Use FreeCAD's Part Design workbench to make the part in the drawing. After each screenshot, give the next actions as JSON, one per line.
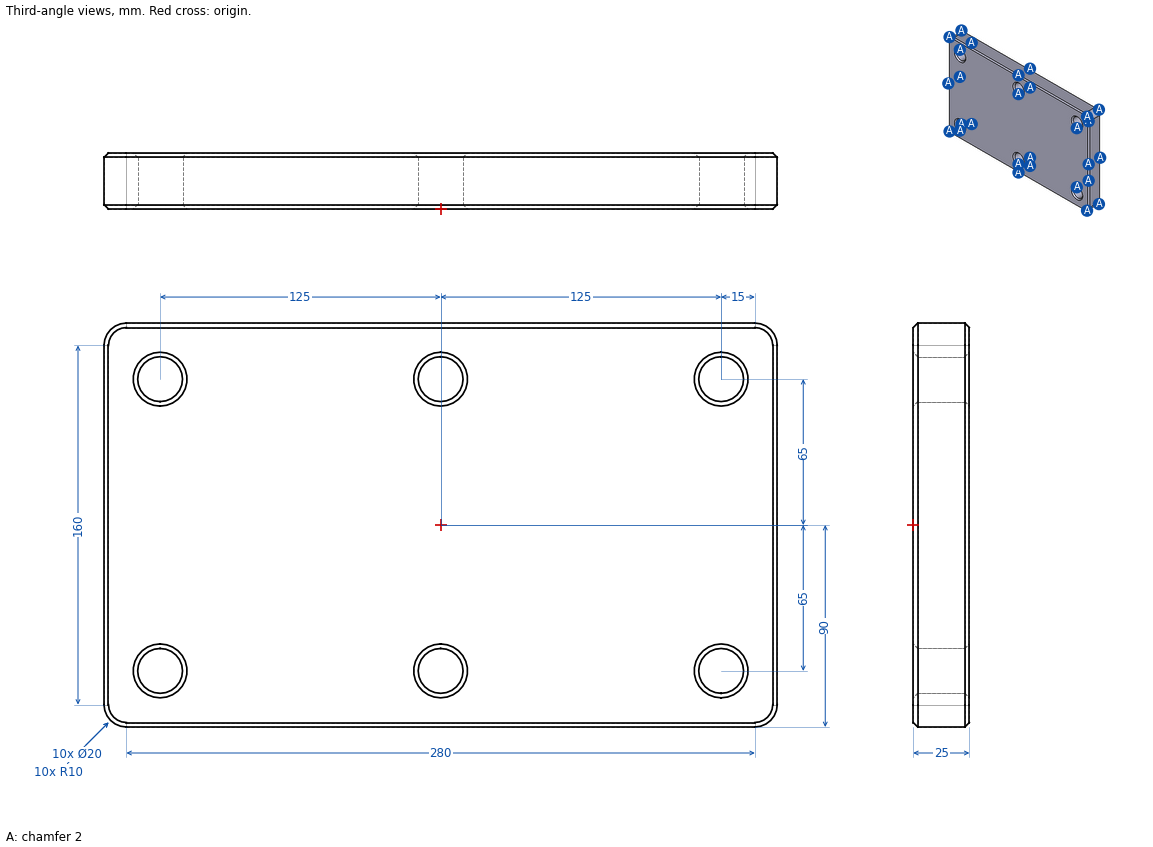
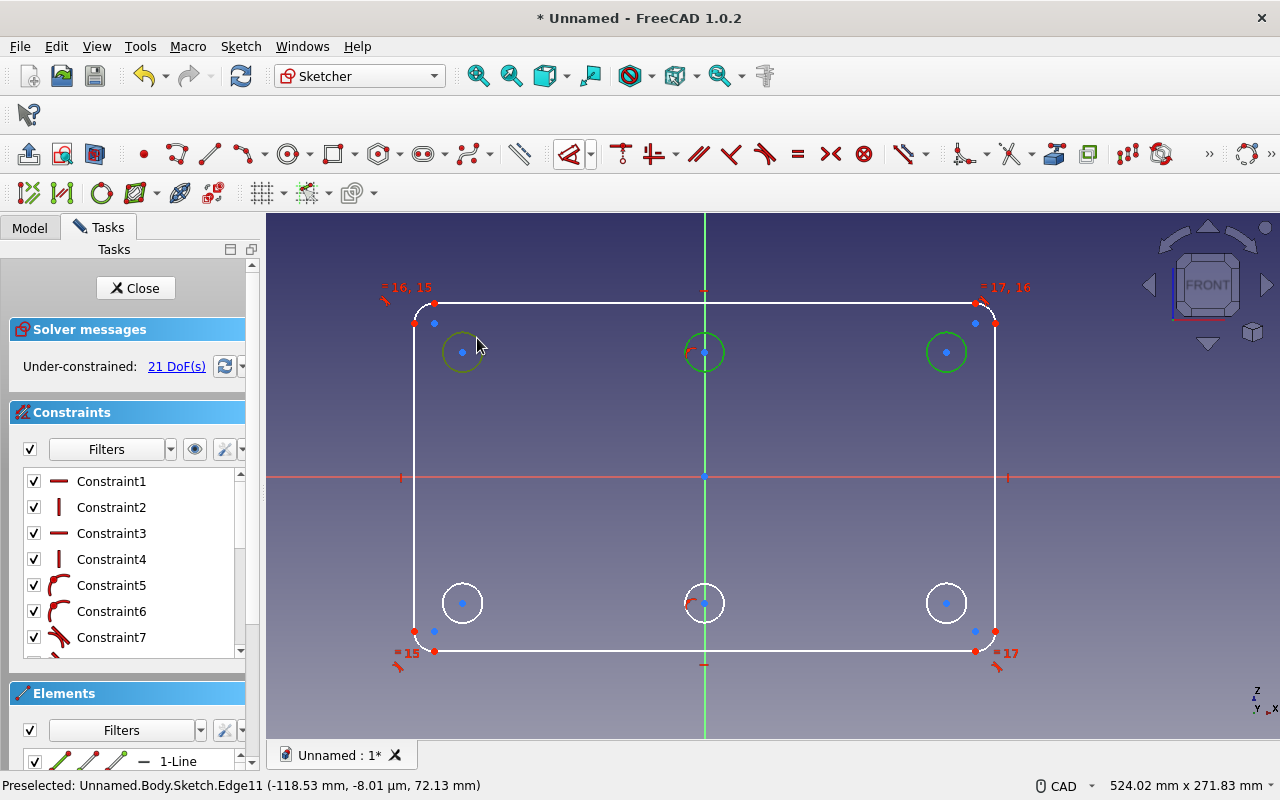
{"action": "left_click", "coordinate": [961, 589]}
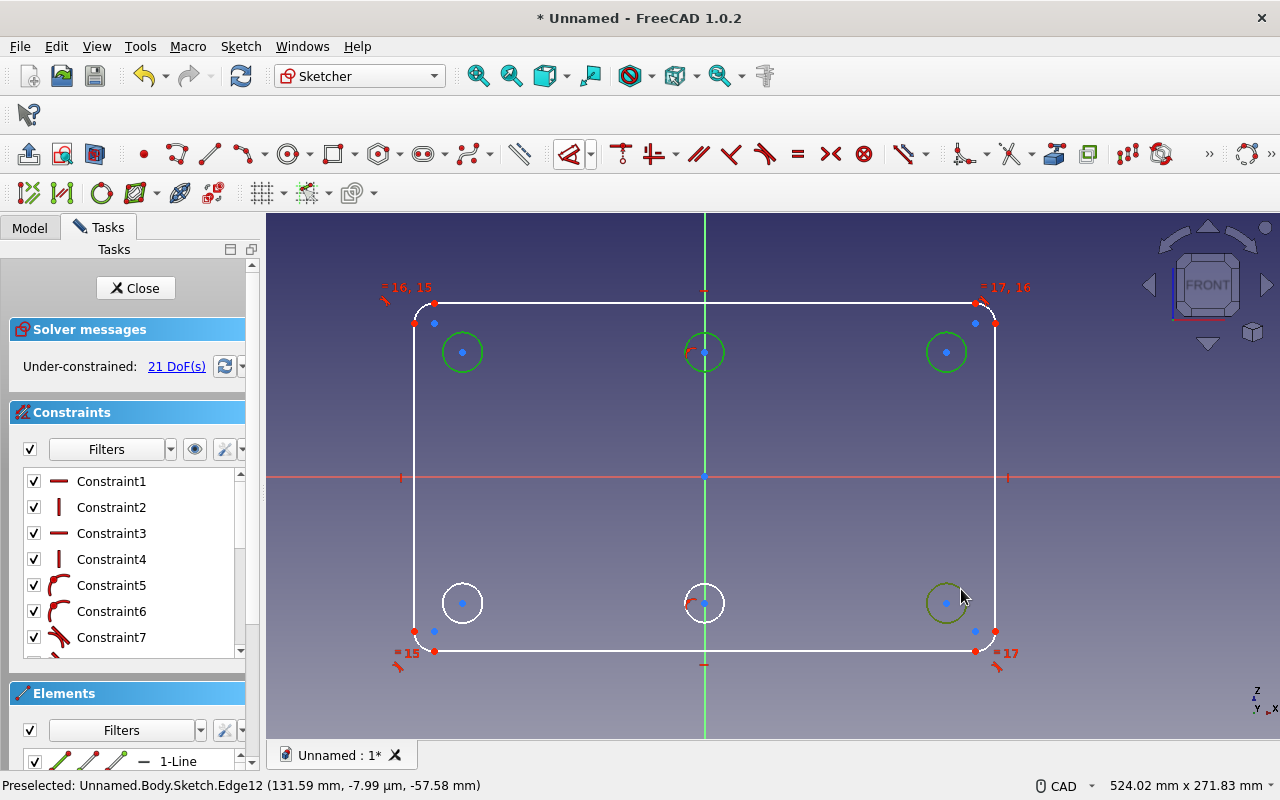
{"action": "left_click", "coordinate": [718, 590]}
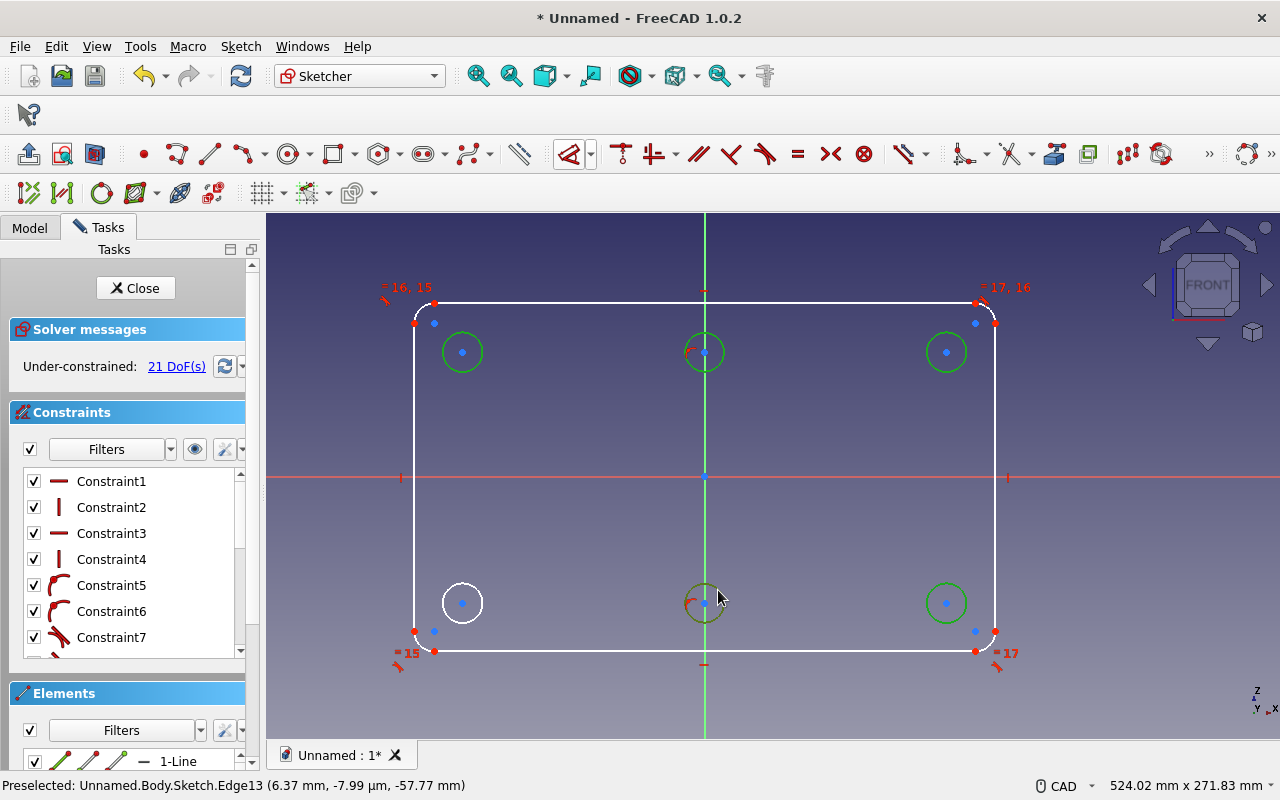
{"action": "left_click", "coordinate": [477, 589]}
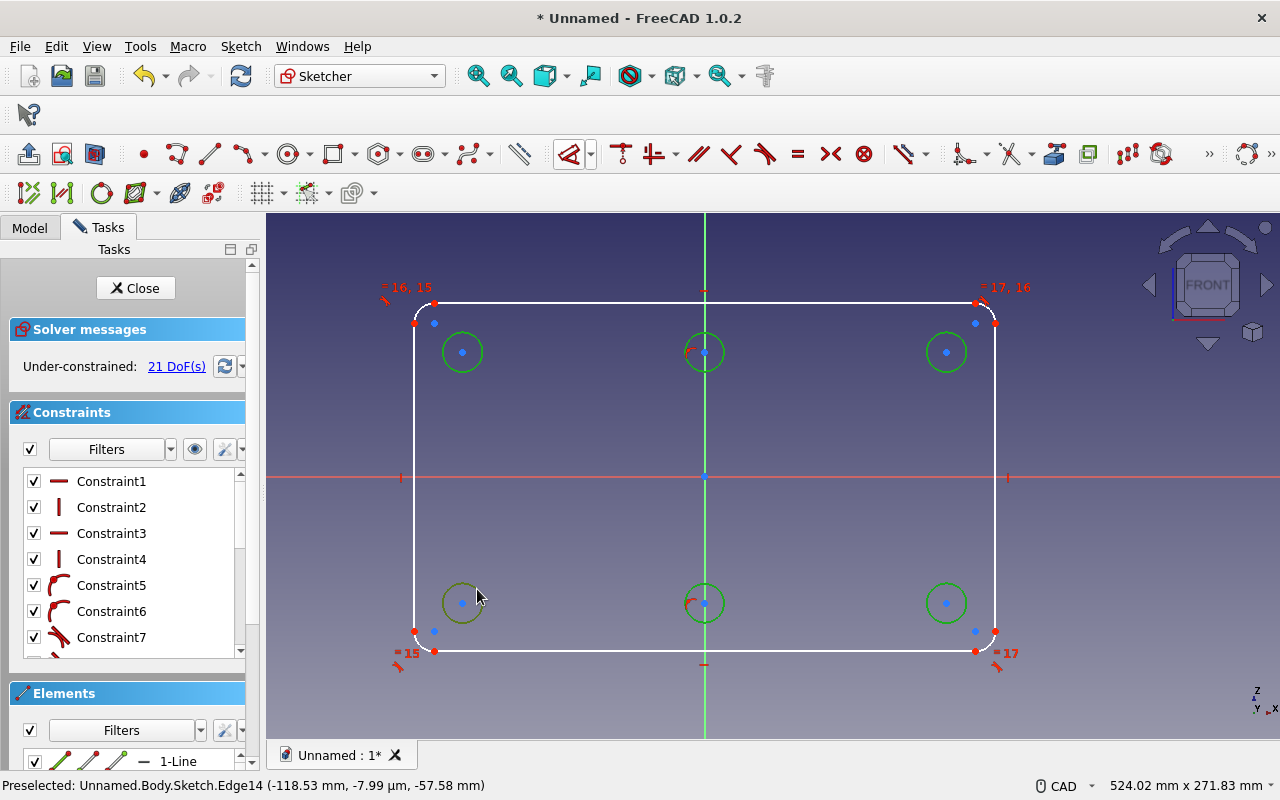
{"action": "left_click", "coordinate": [798, 154]}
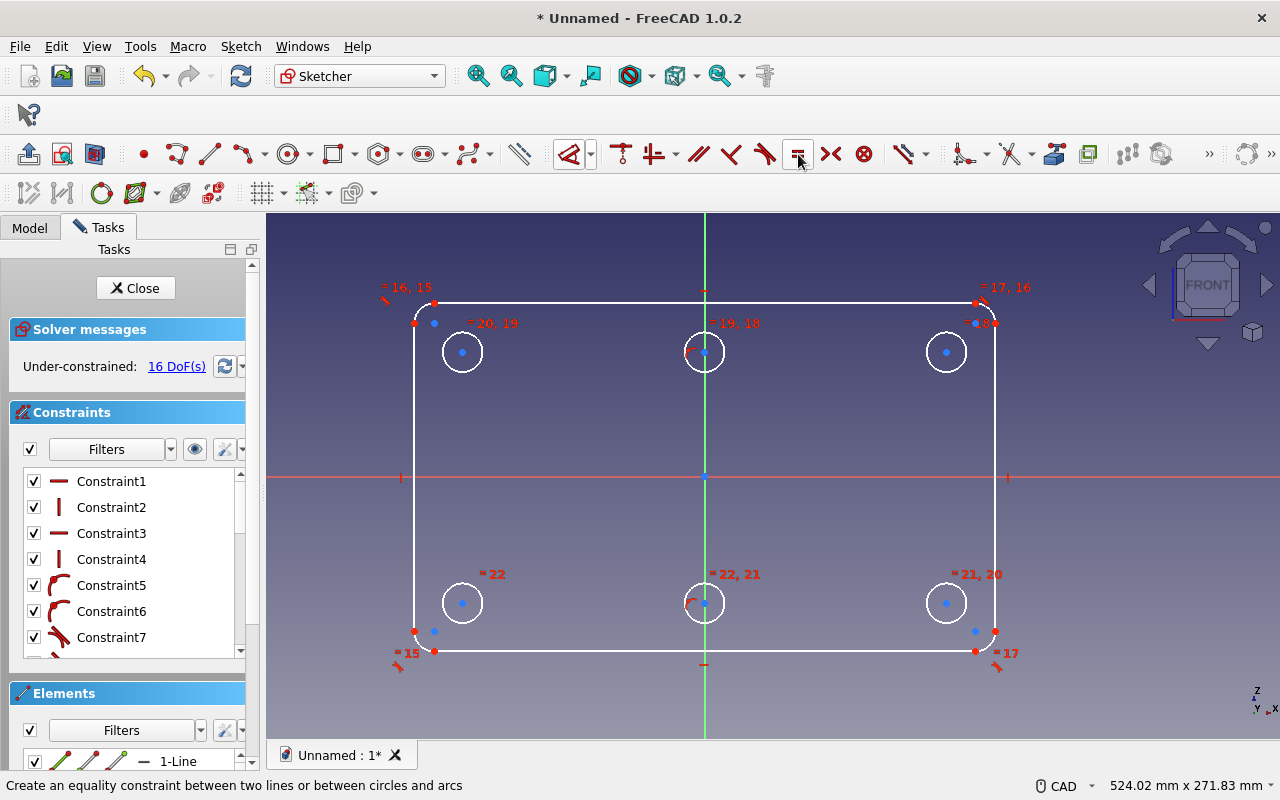
{"action": "left_click", "coordinate": [947, 352]}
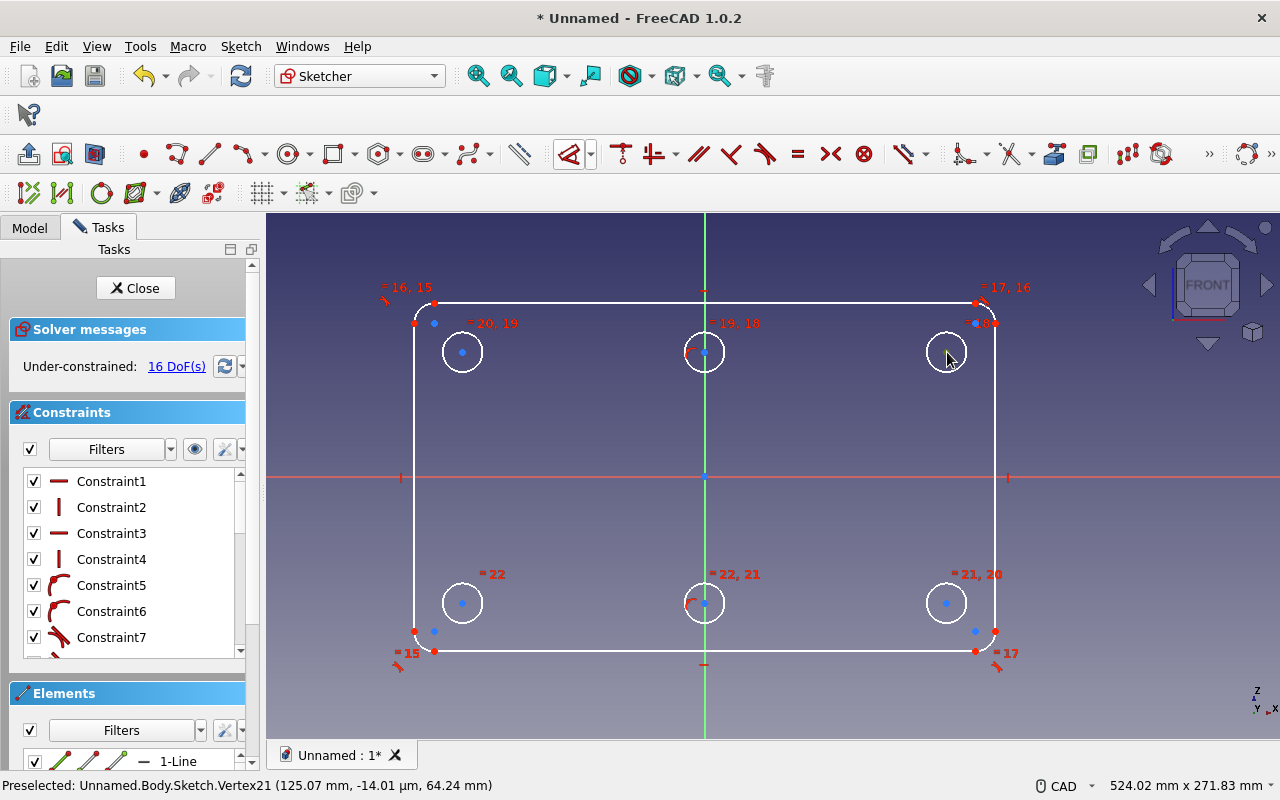
{"action": "left_click", "coordinate": [705, 352]}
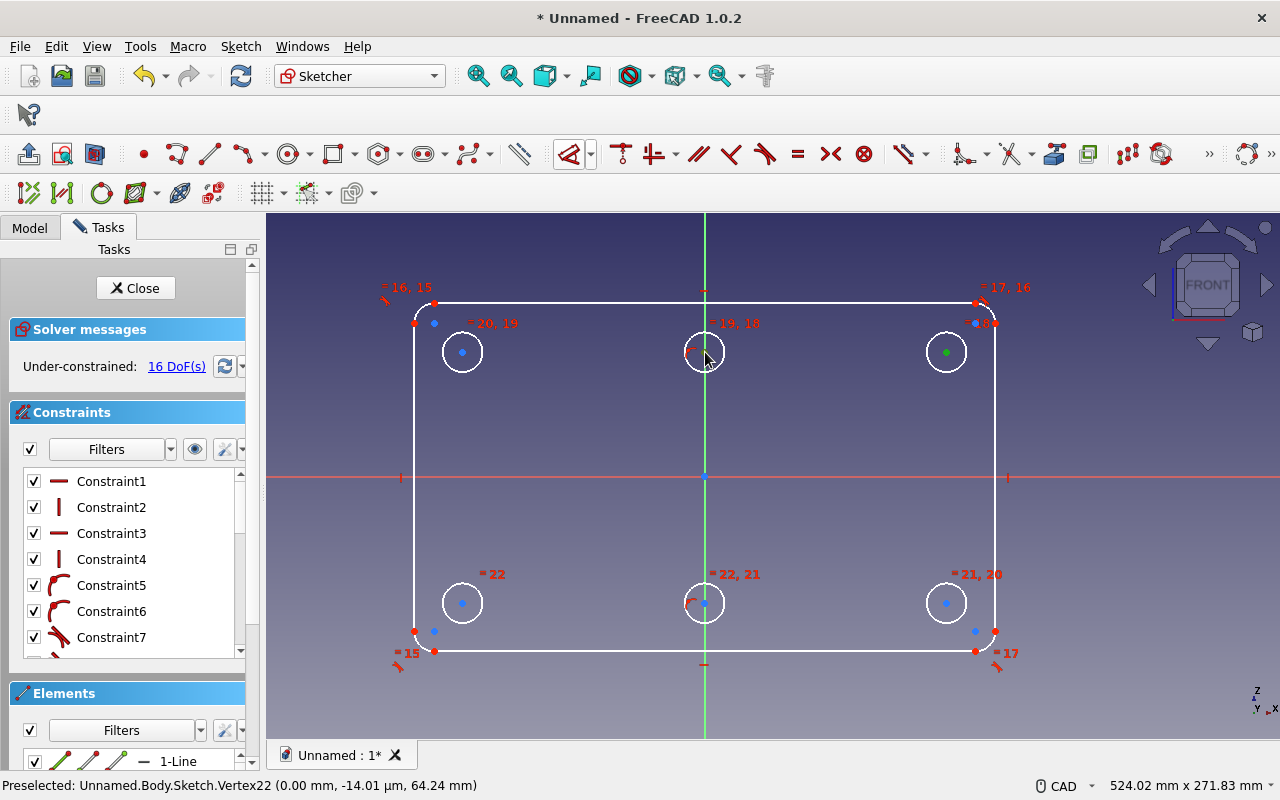
{"action": "left_click", "coordinate": [676, 154]}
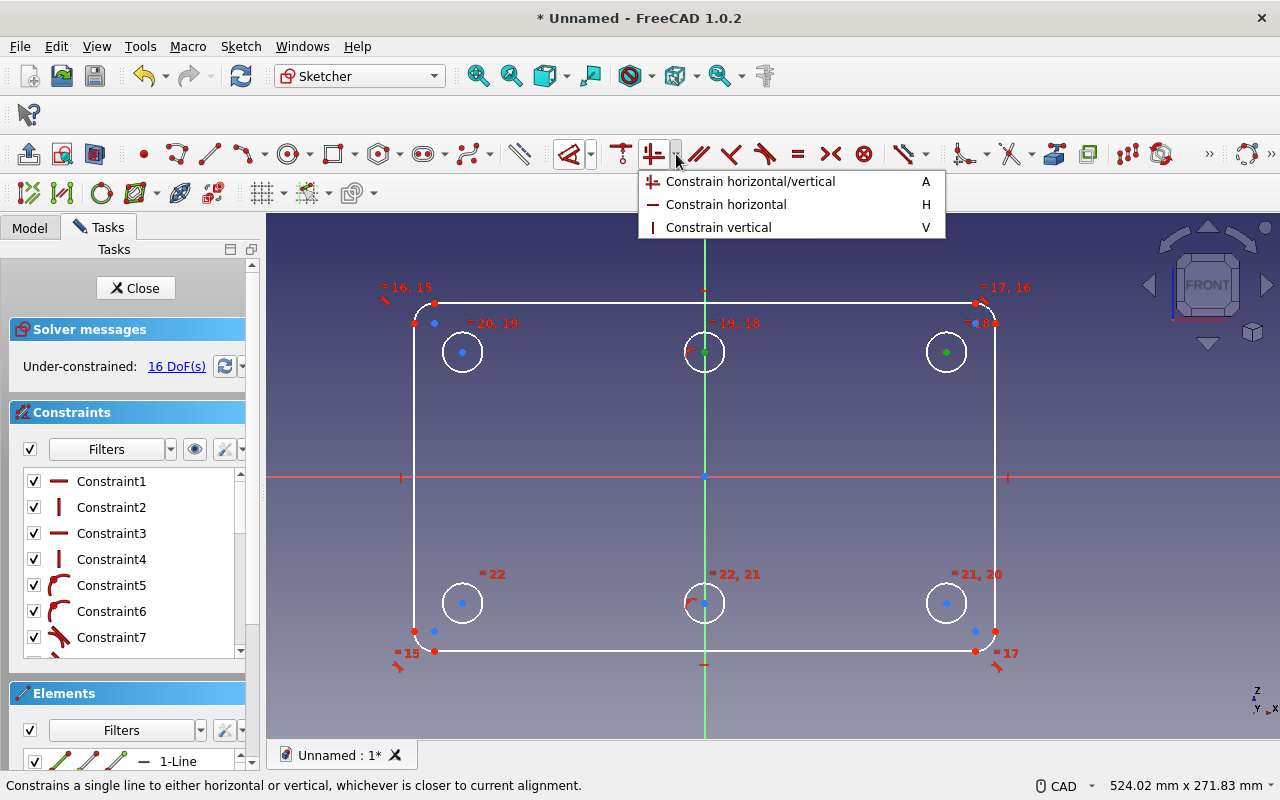
{"action": "left_click", "coordinate": [792, 204]}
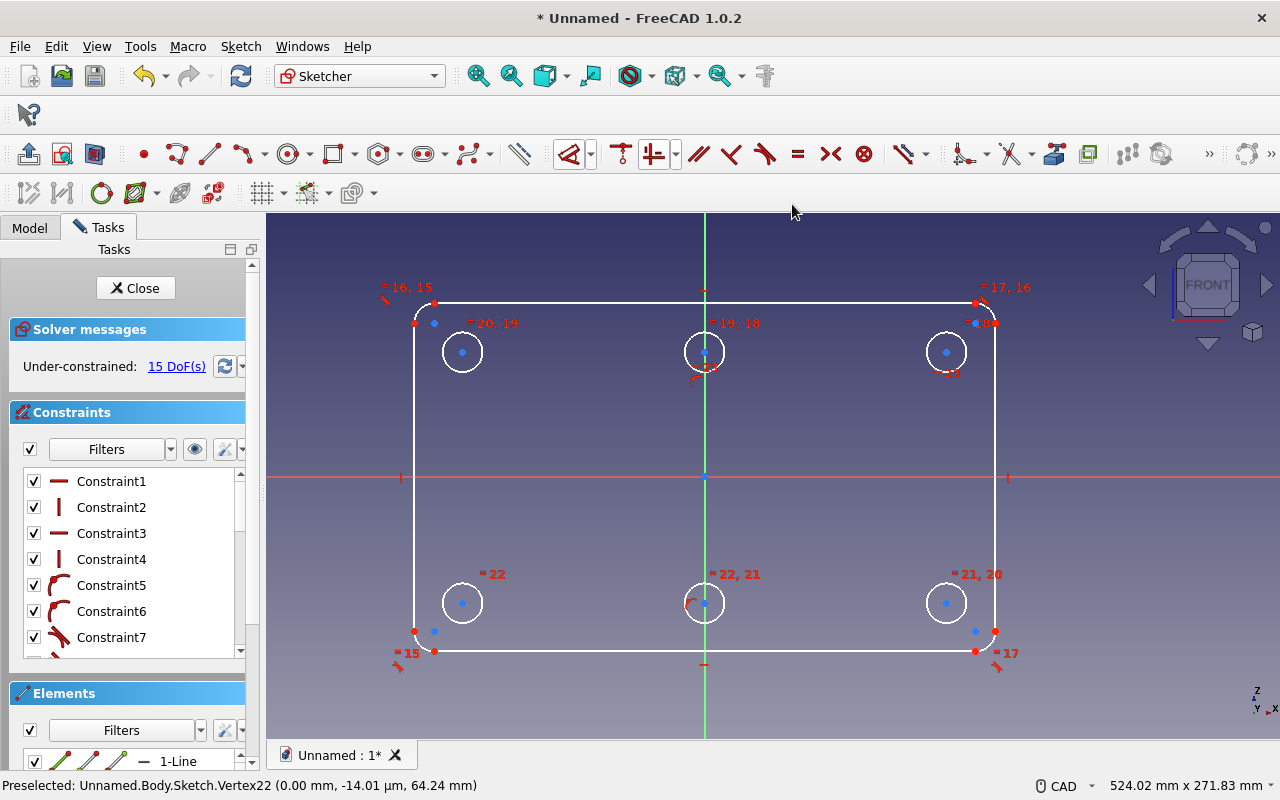
{"action": "left_click", "coordinate": [705, 352]}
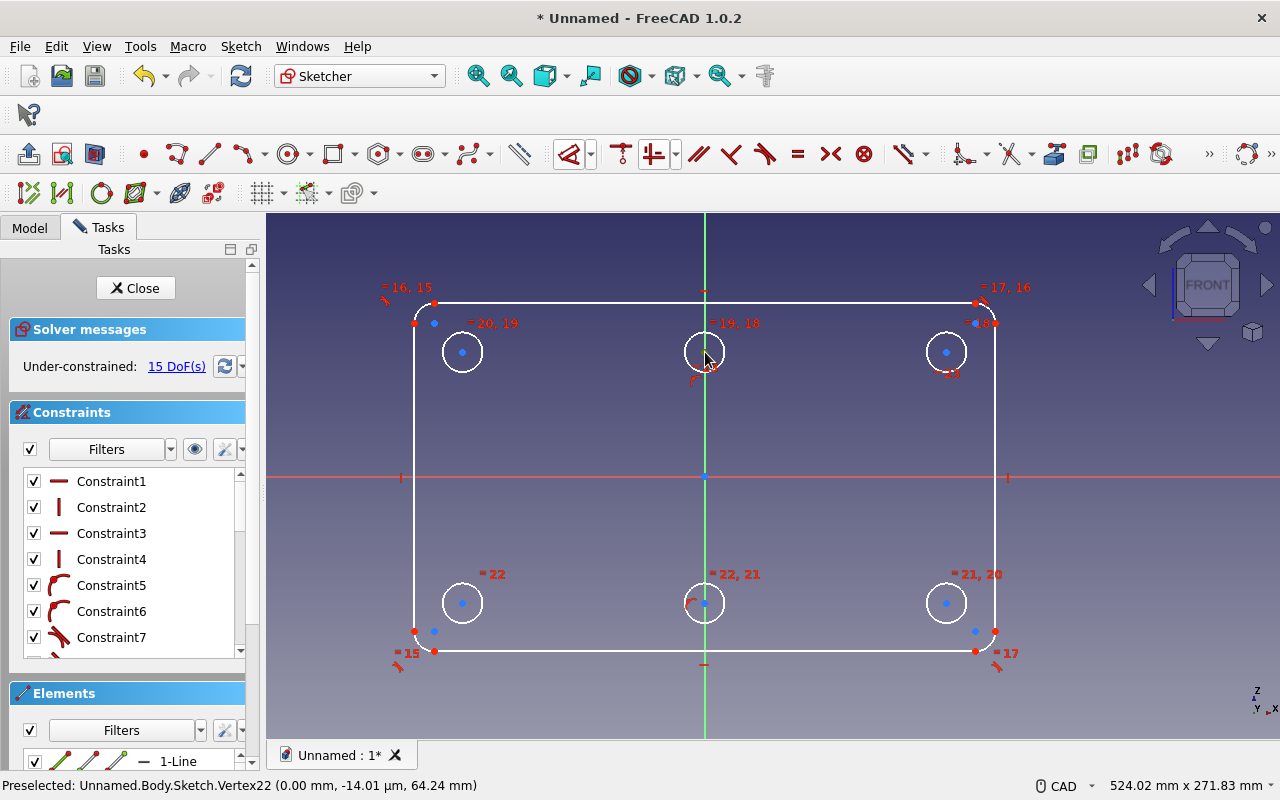
{"action": "left_click", "coordinate": [463, 352]}